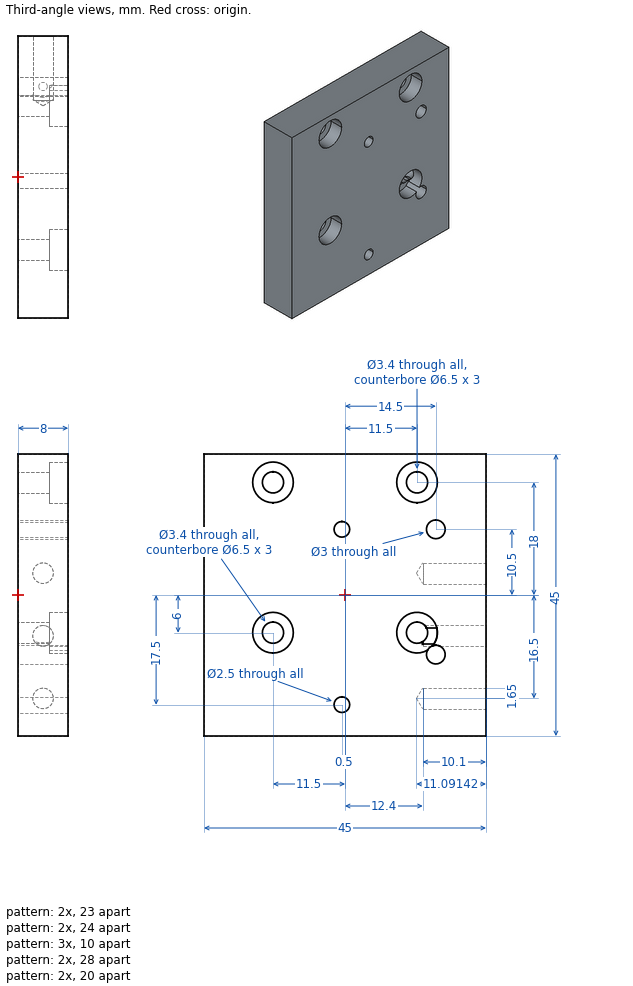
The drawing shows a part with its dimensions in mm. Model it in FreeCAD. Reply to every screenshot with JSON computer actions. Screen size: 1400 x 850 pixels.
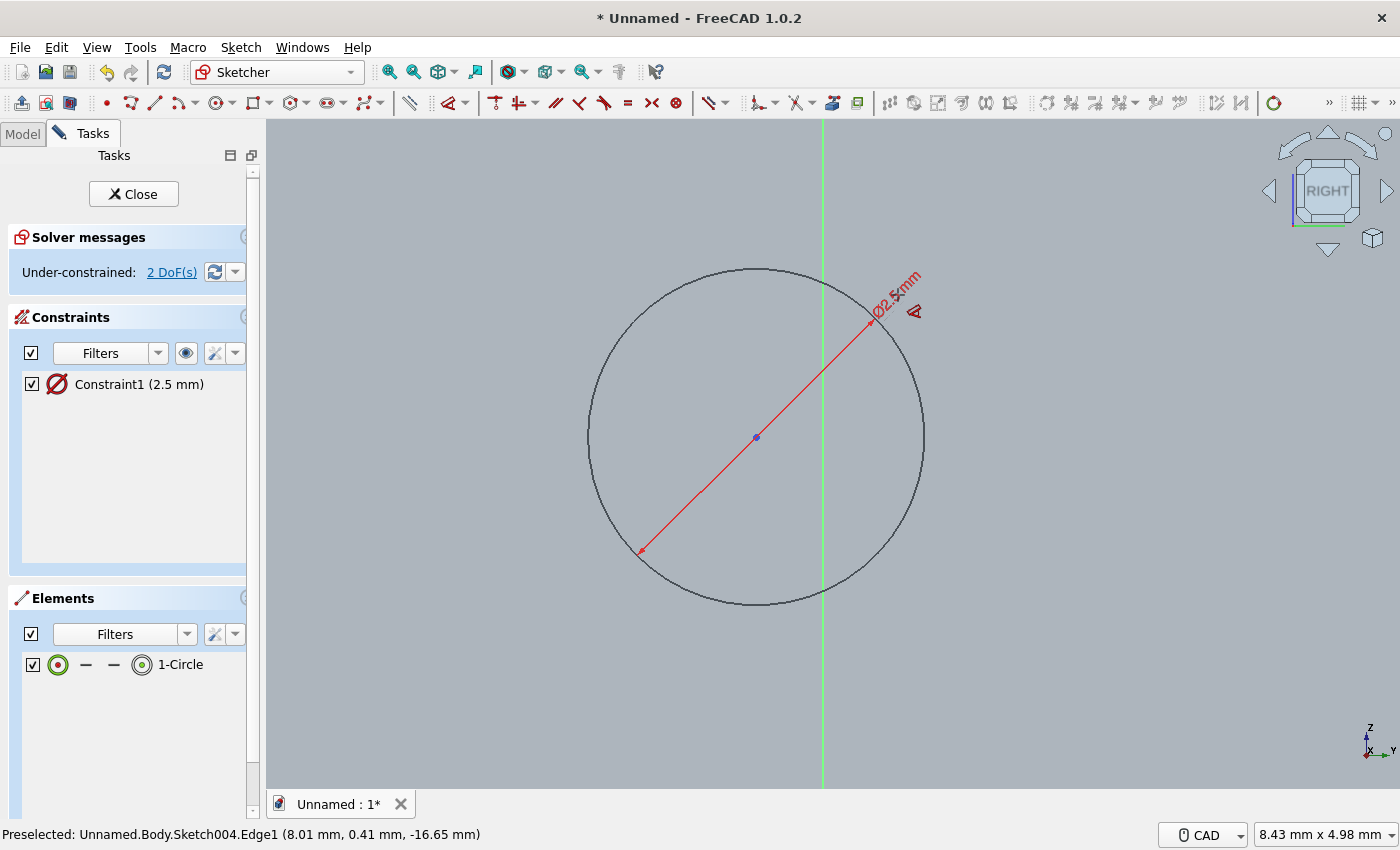
{"action": "left_click", "coordinate": [756, 437]}
{"action": "left_click", "coordinate": [790, 471]}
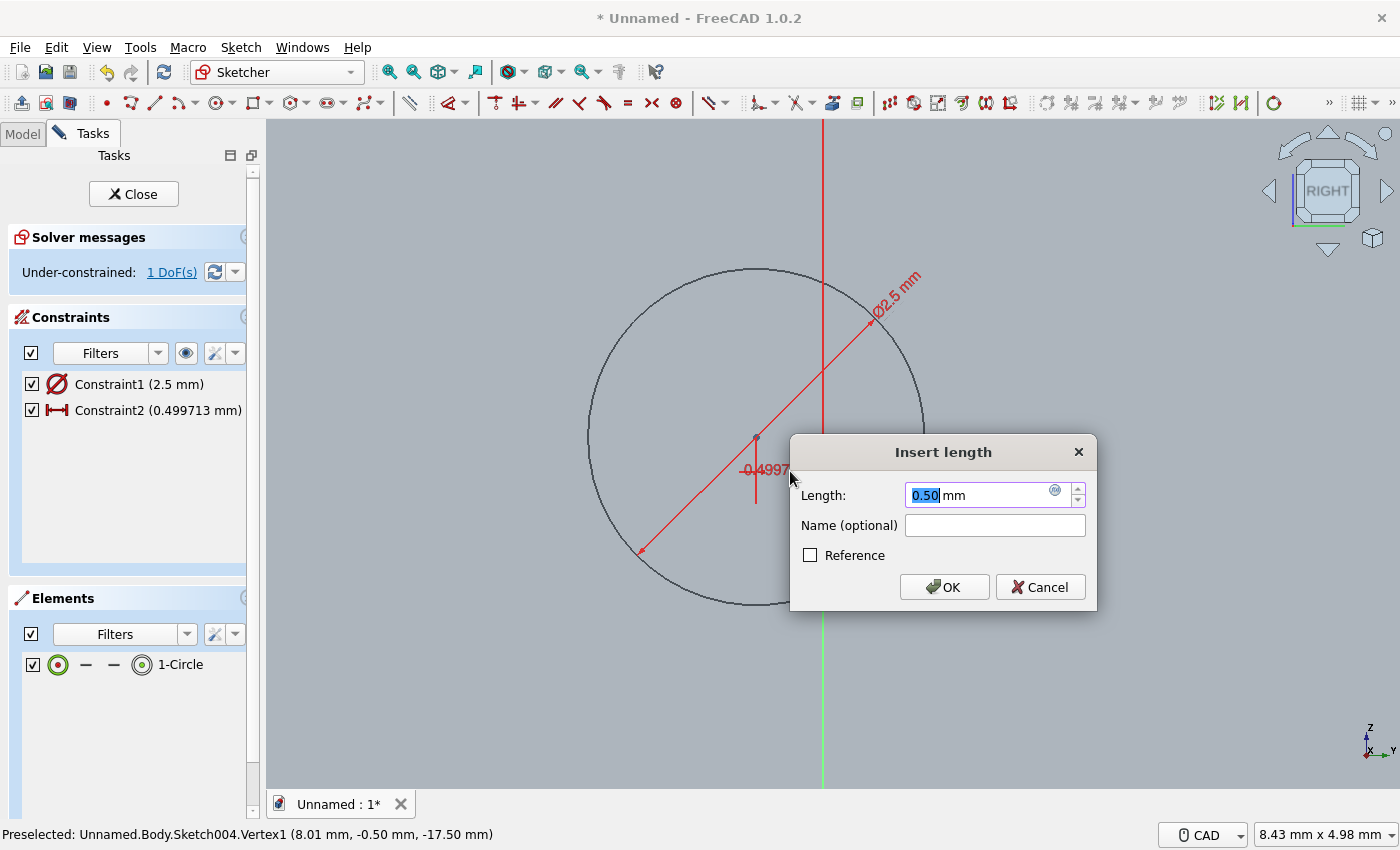
{"action": "type", "text": "0.5"}
{"action": "key", "text": "Return"}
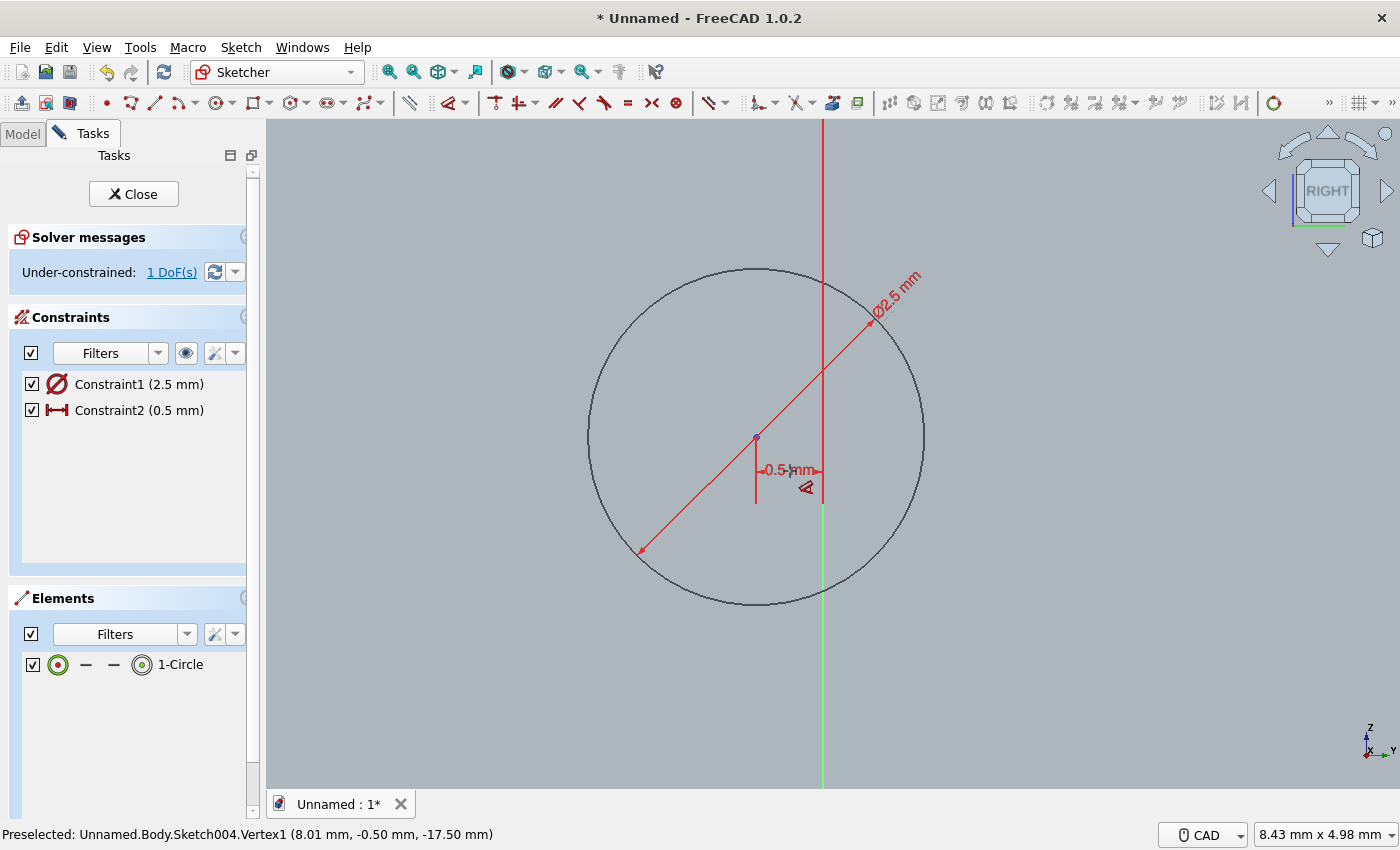
{"action": "left_click", "coordinate": [756, 437]}
{"action": "left_click", "coordinate": [857, 225]}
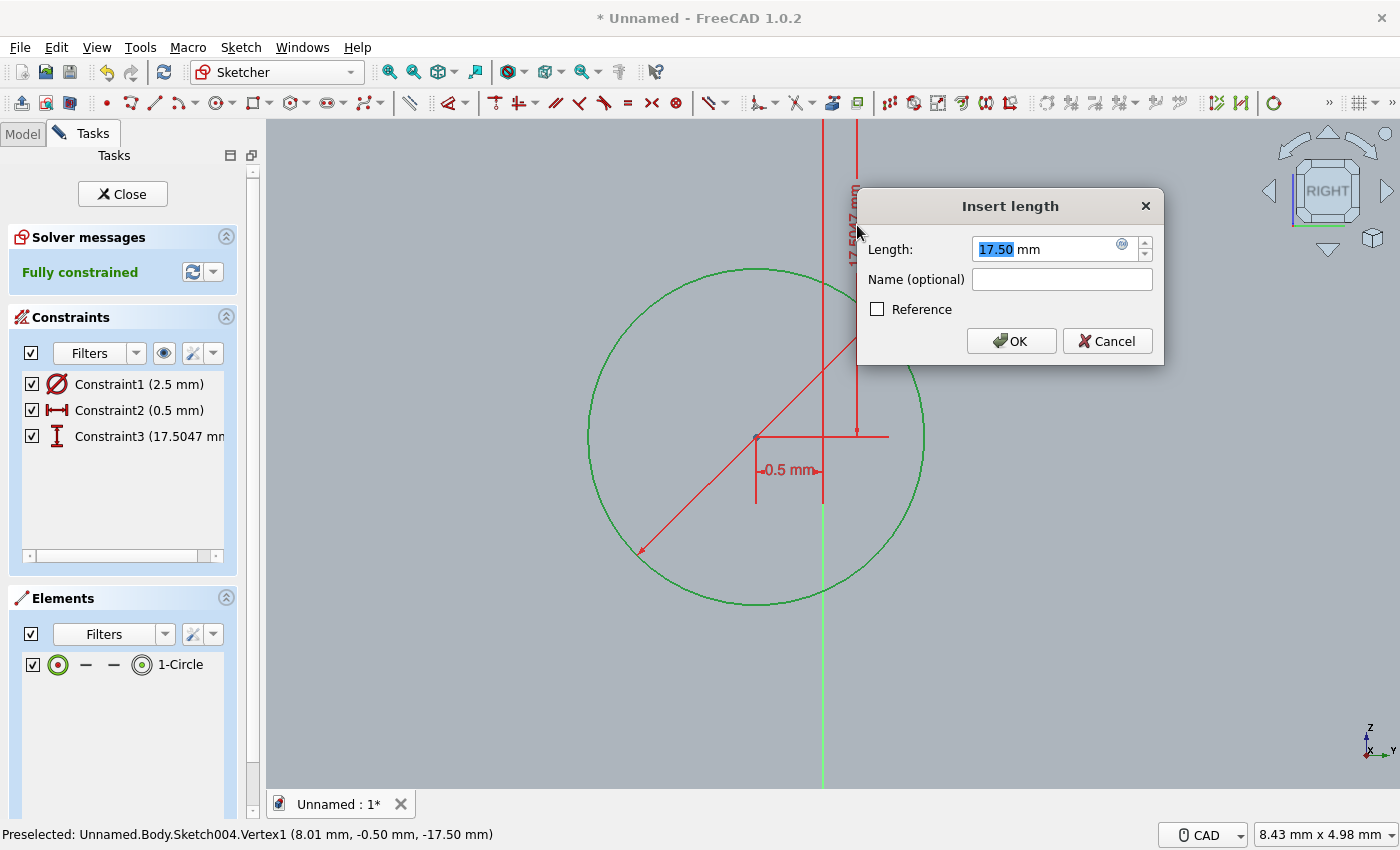
{"action": "type", "text": "17.5"}
{"action": "key", "text": "Return"}
{"action": "key", "text": "Escape"}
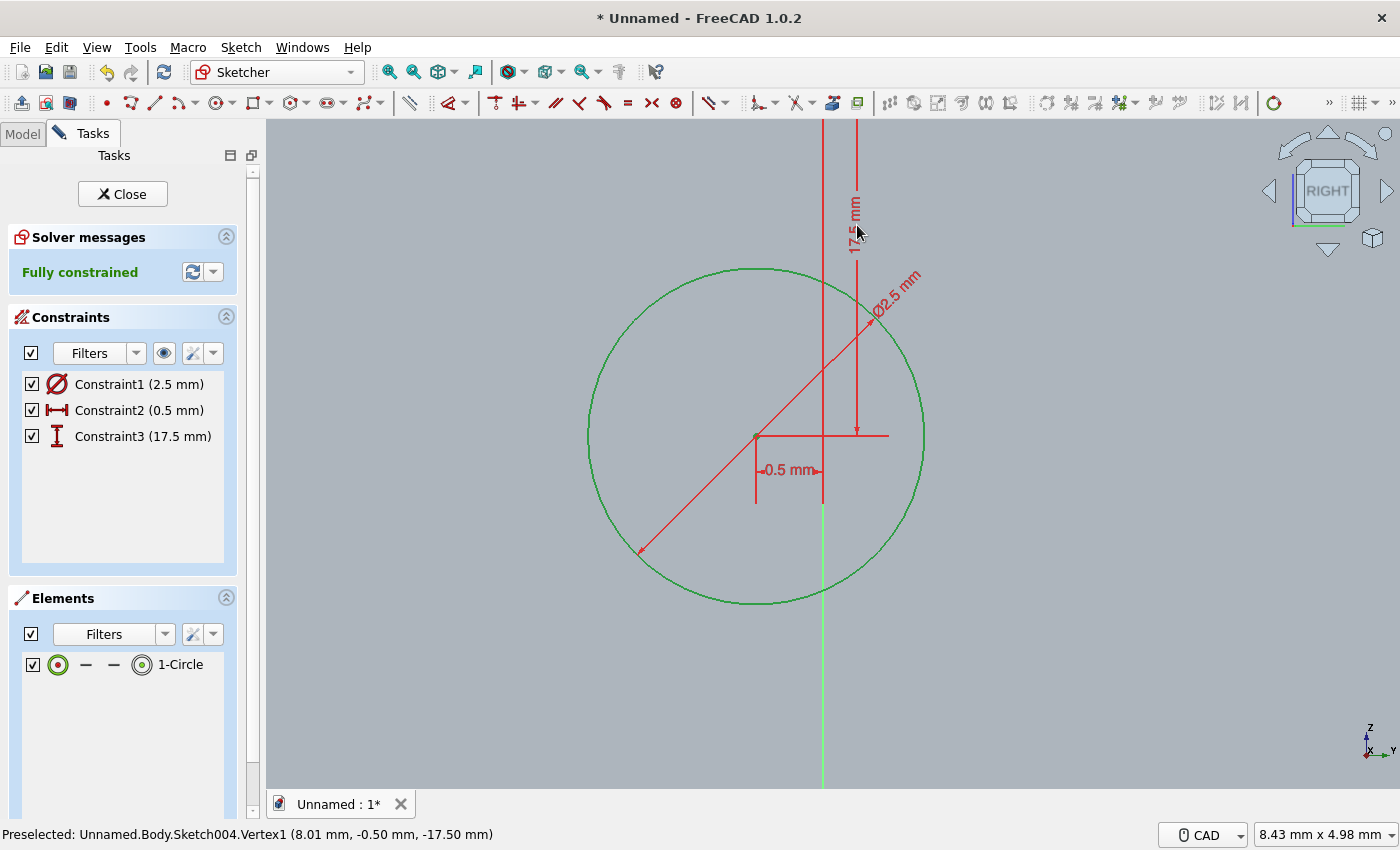
{"action": "left_click", "coordinate": [123, 194]}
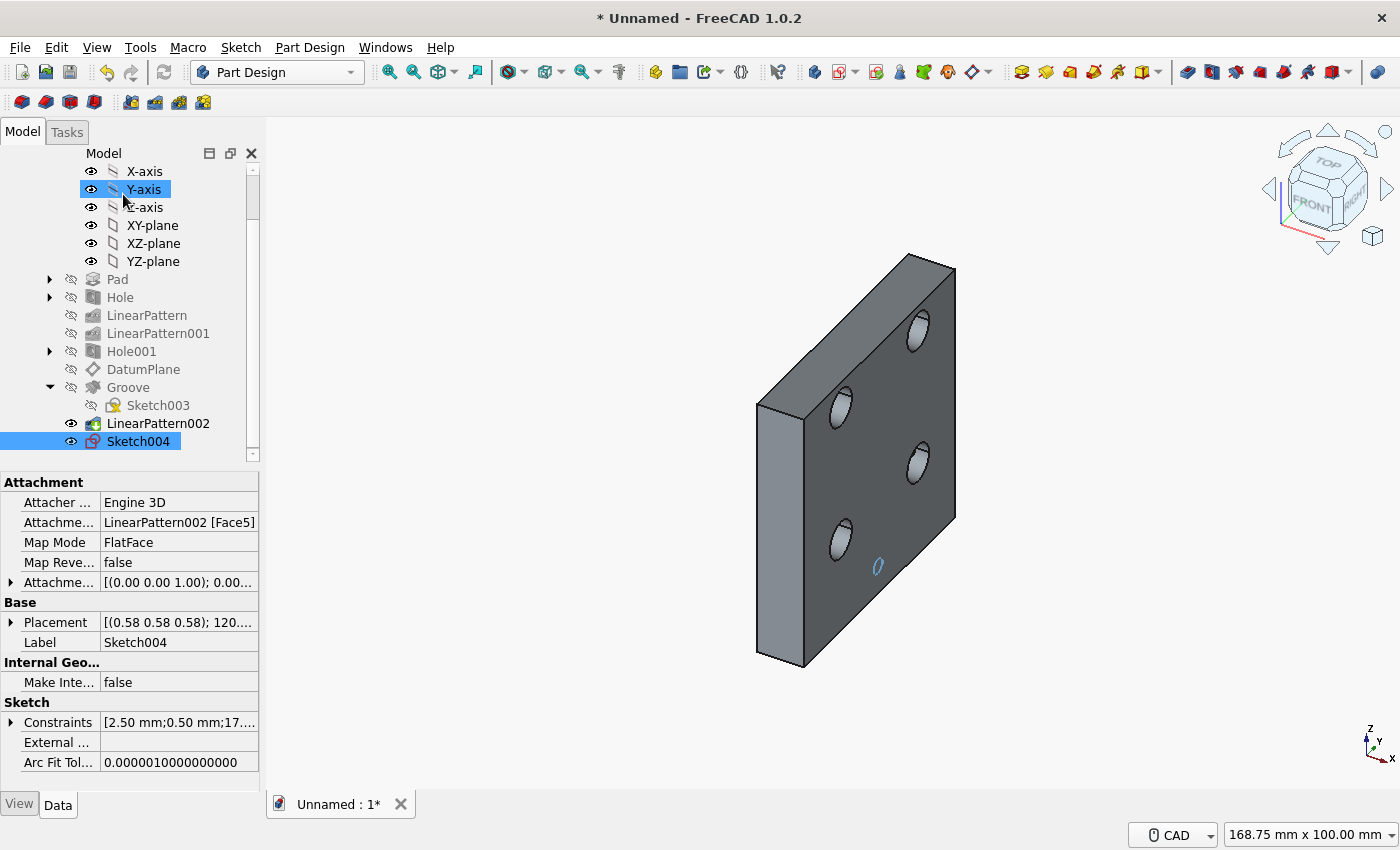
{"action": "left_click", "coordinate": [1212, 72]}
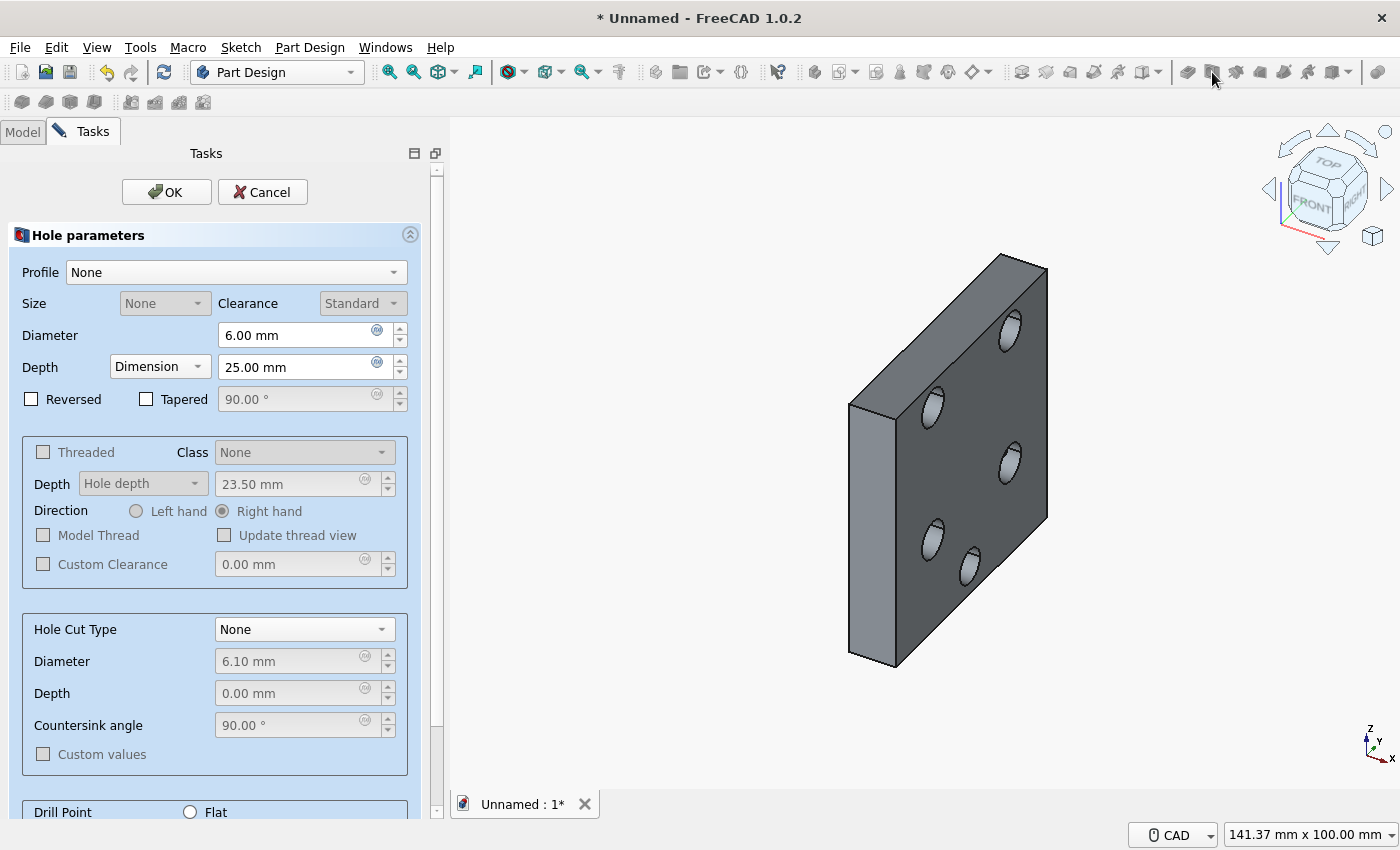
{"action": "triple_click", "coordinate": [305, 335]}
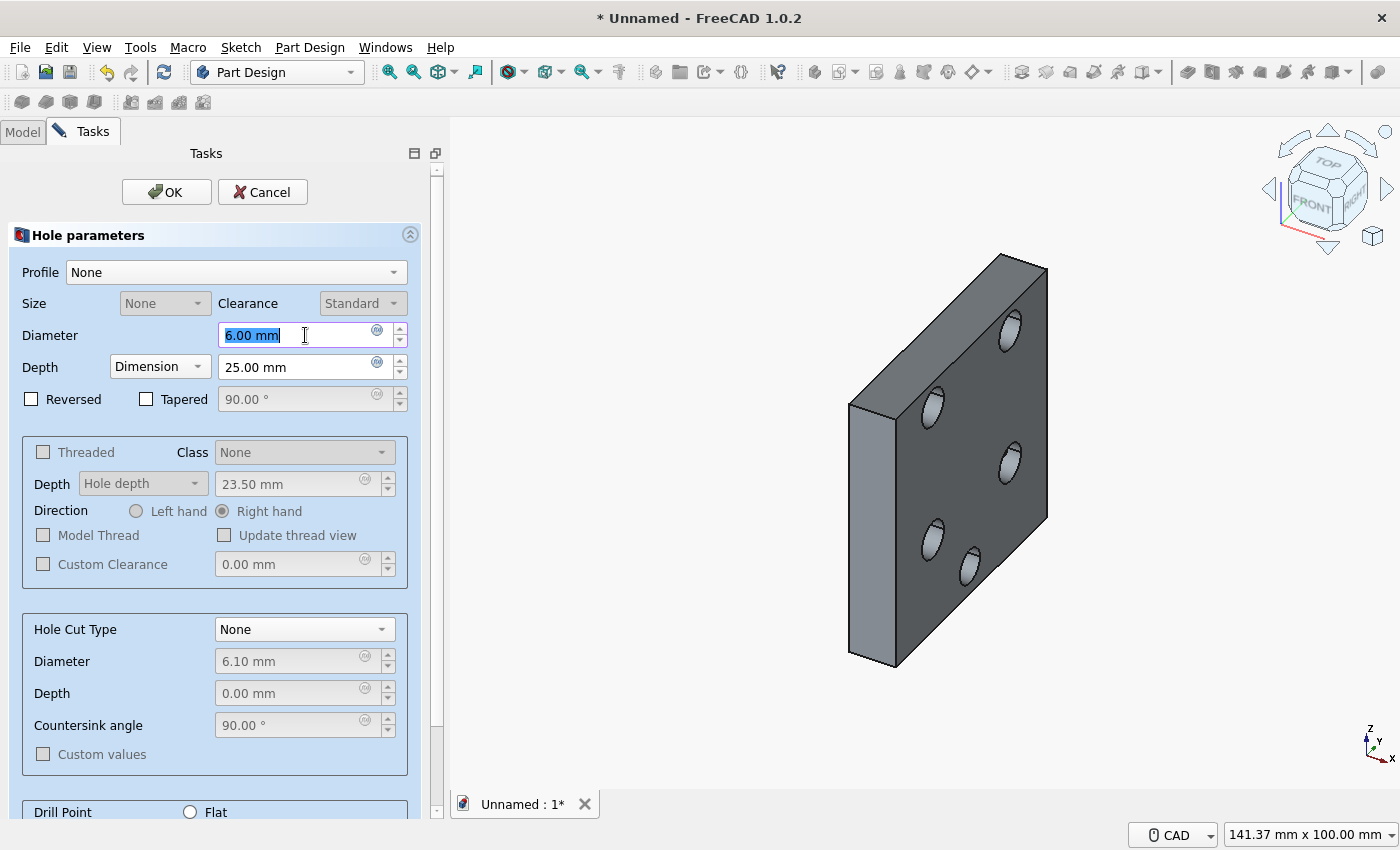
{"action": "type", "text": "2.5"}
{"action": "key", "text": "Tab"}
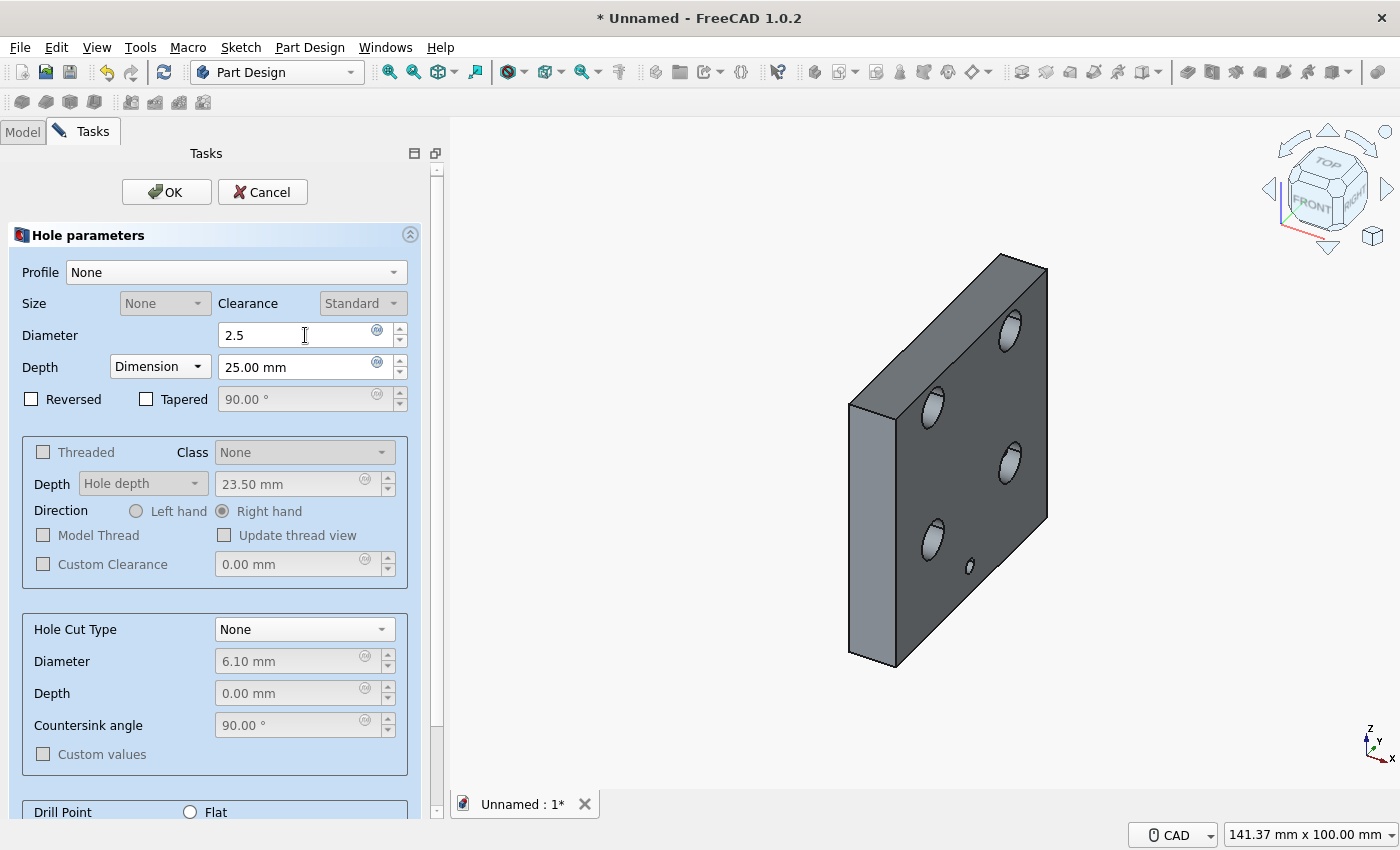
{"action": "left_click", "coordinate": [161, 366]}